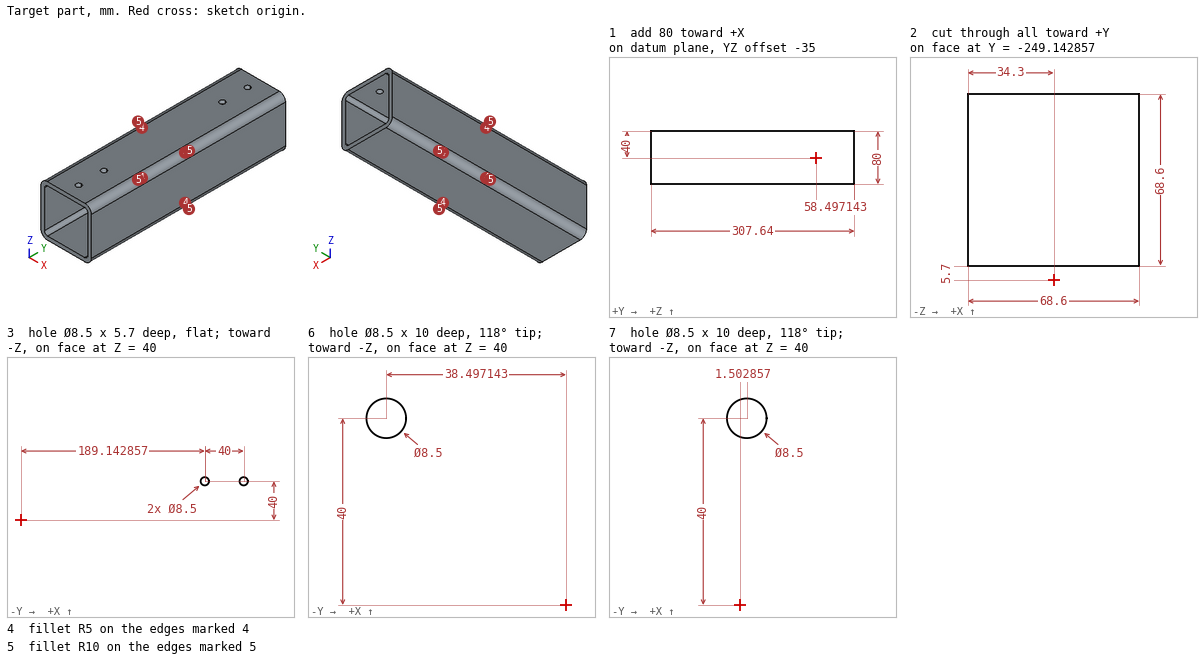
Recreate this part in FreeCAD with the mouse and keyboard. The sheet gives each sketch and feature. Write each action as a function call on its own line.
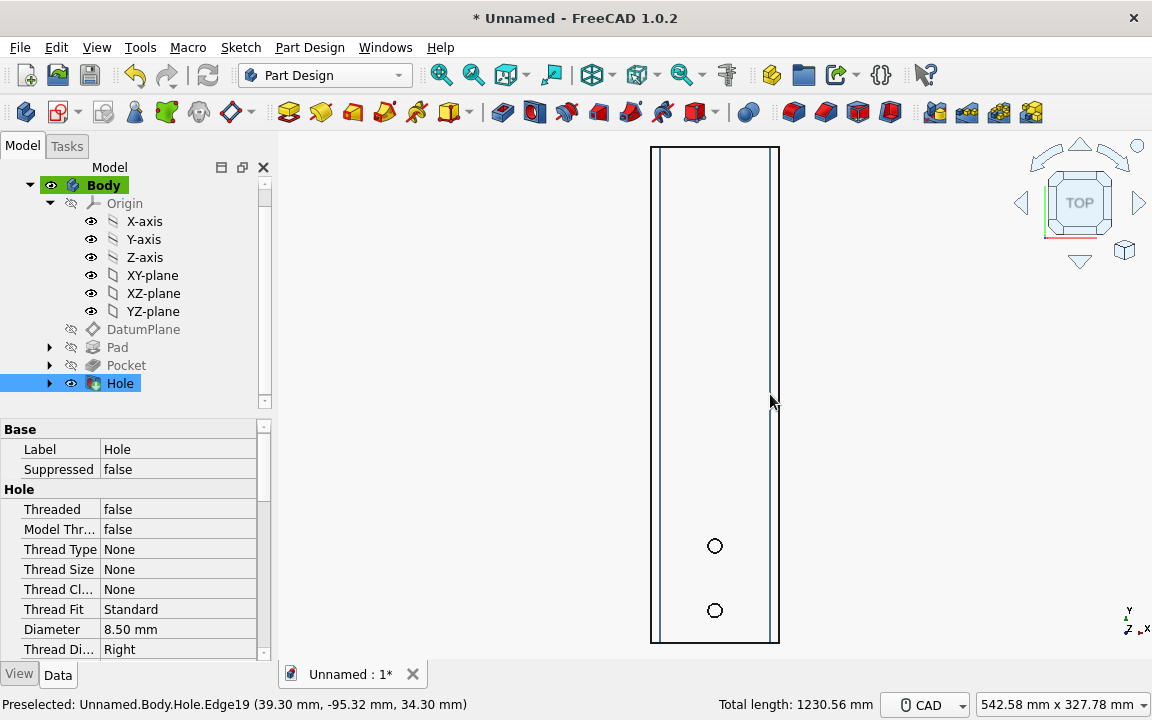
key(v)
key(1)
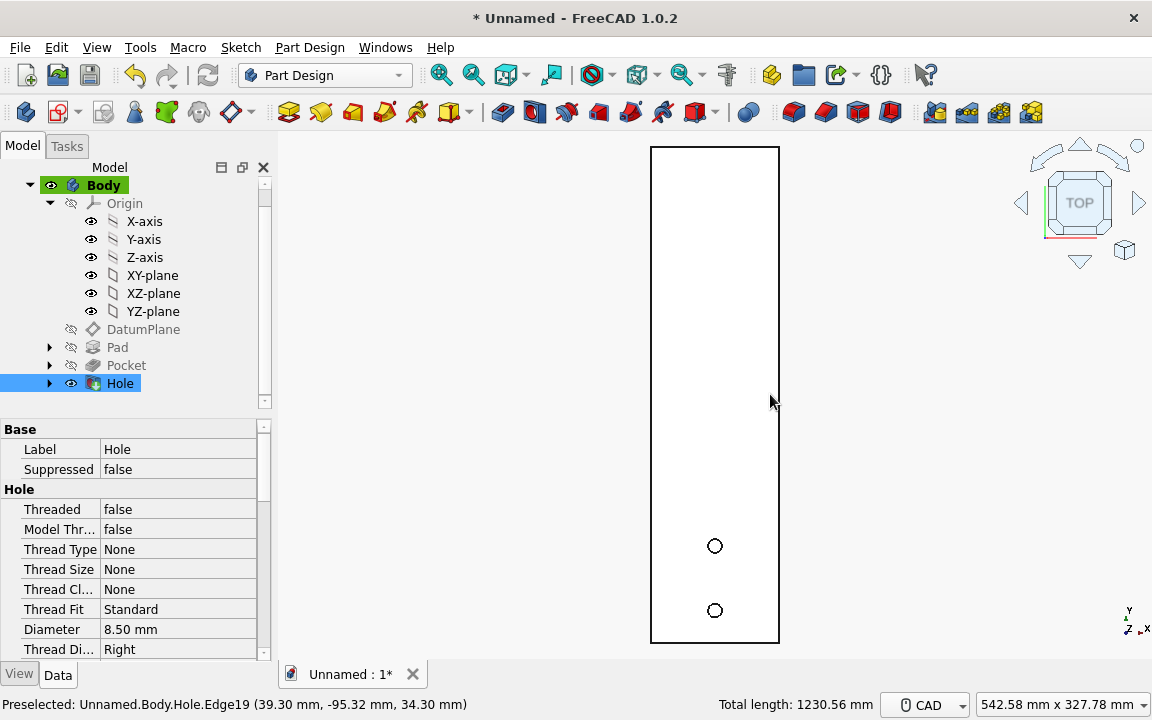
click(794, 112)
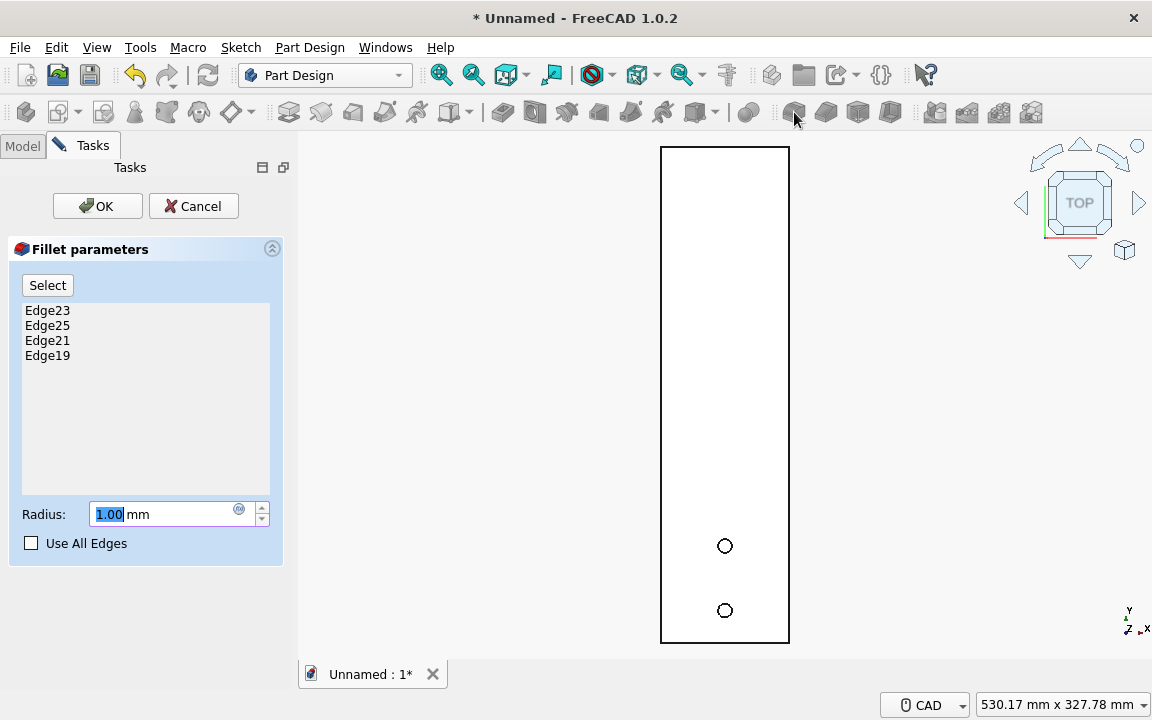
text(5)
key(Tab)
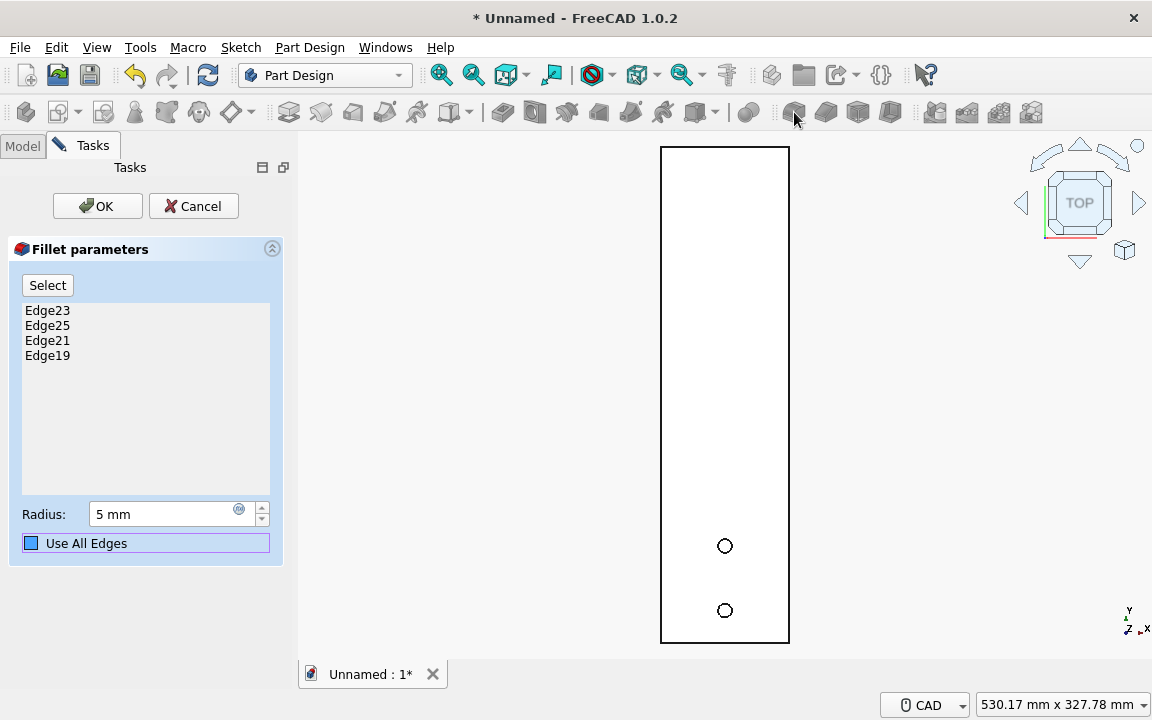
click(98, 206)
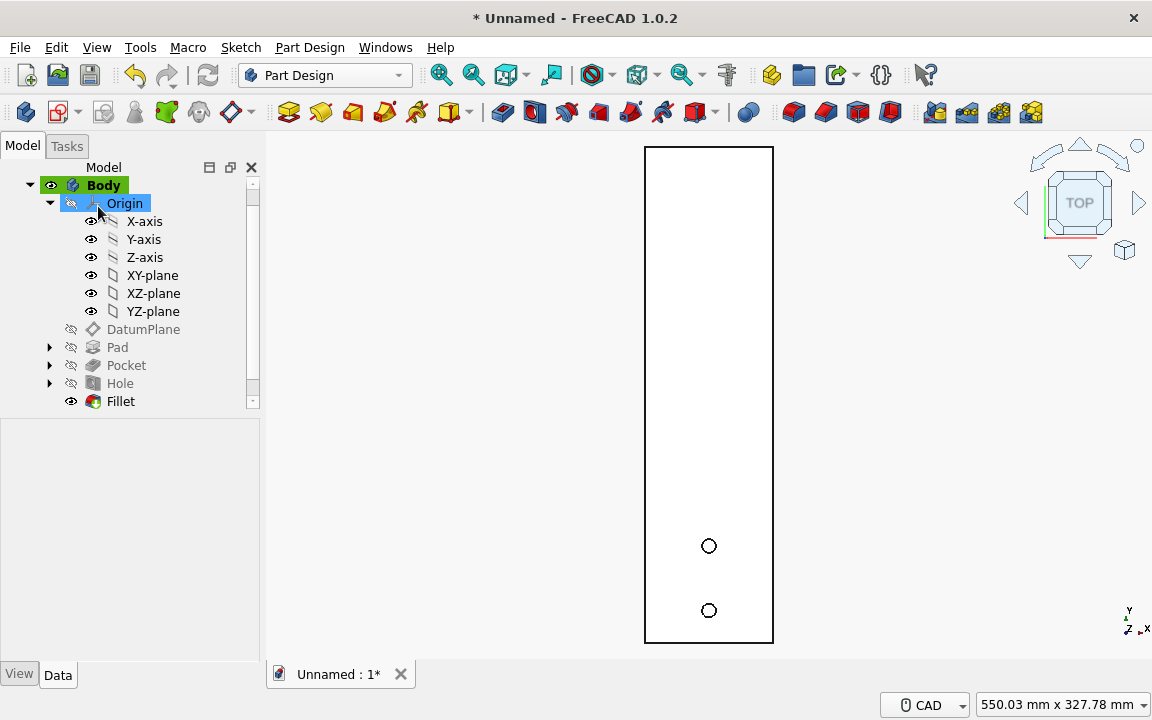
click(773, 394)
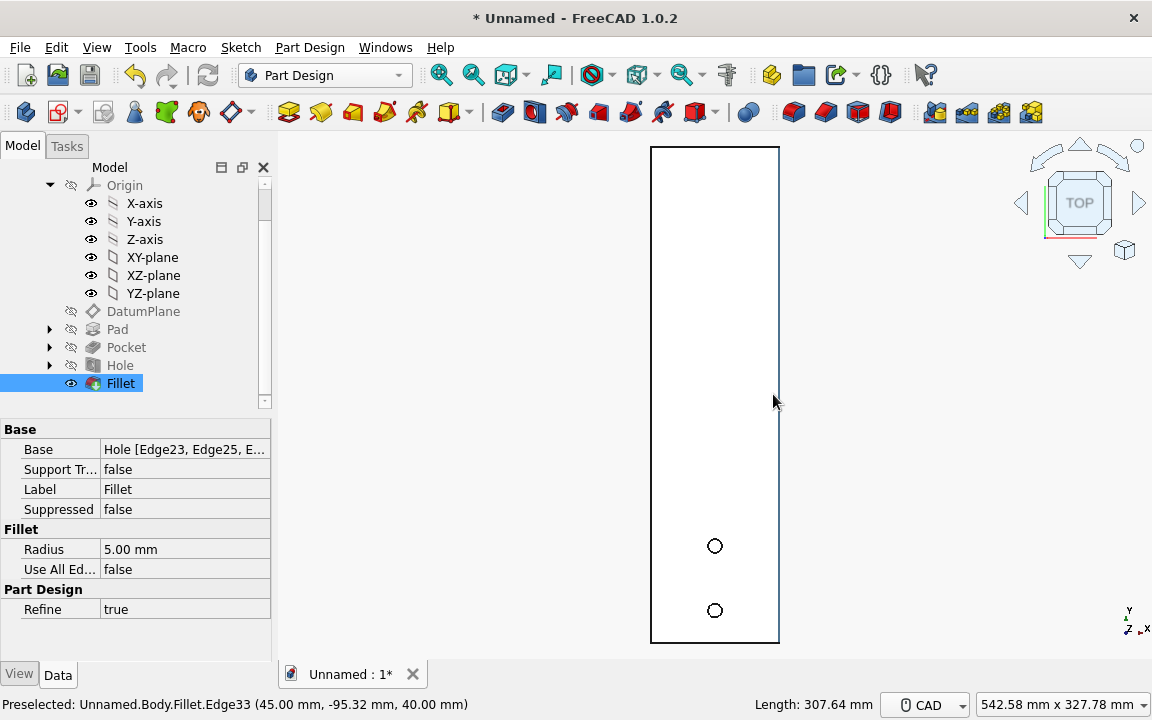
click(651, 394, ctrl)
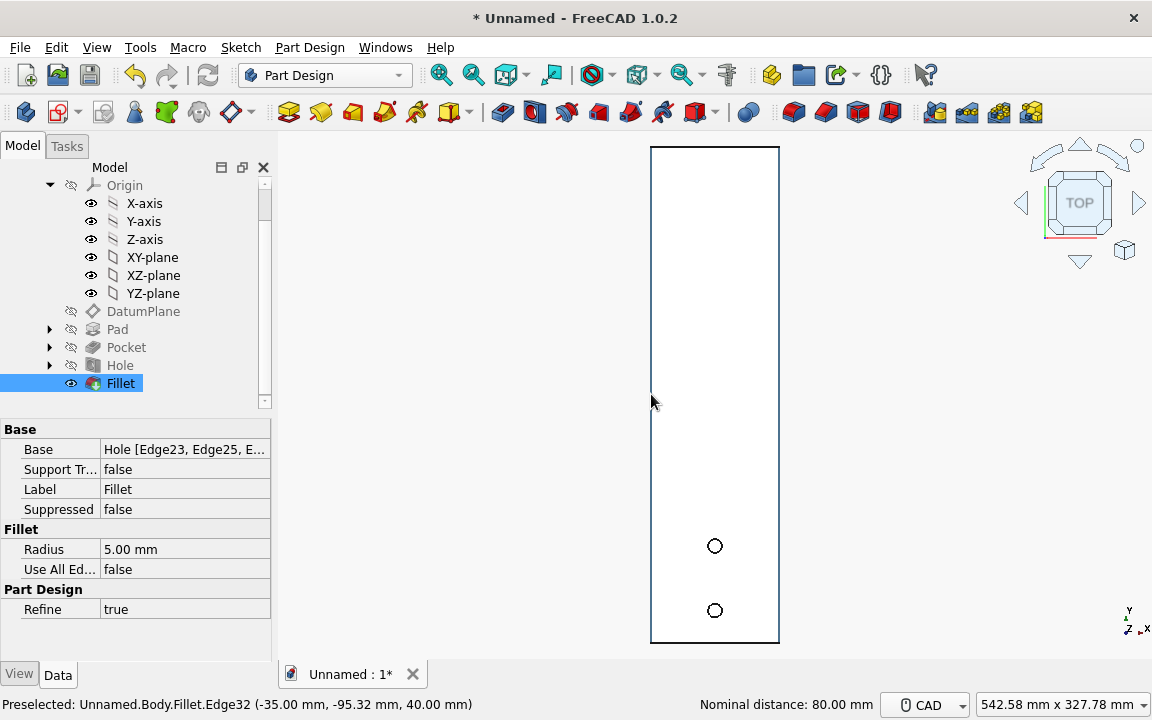
key(0)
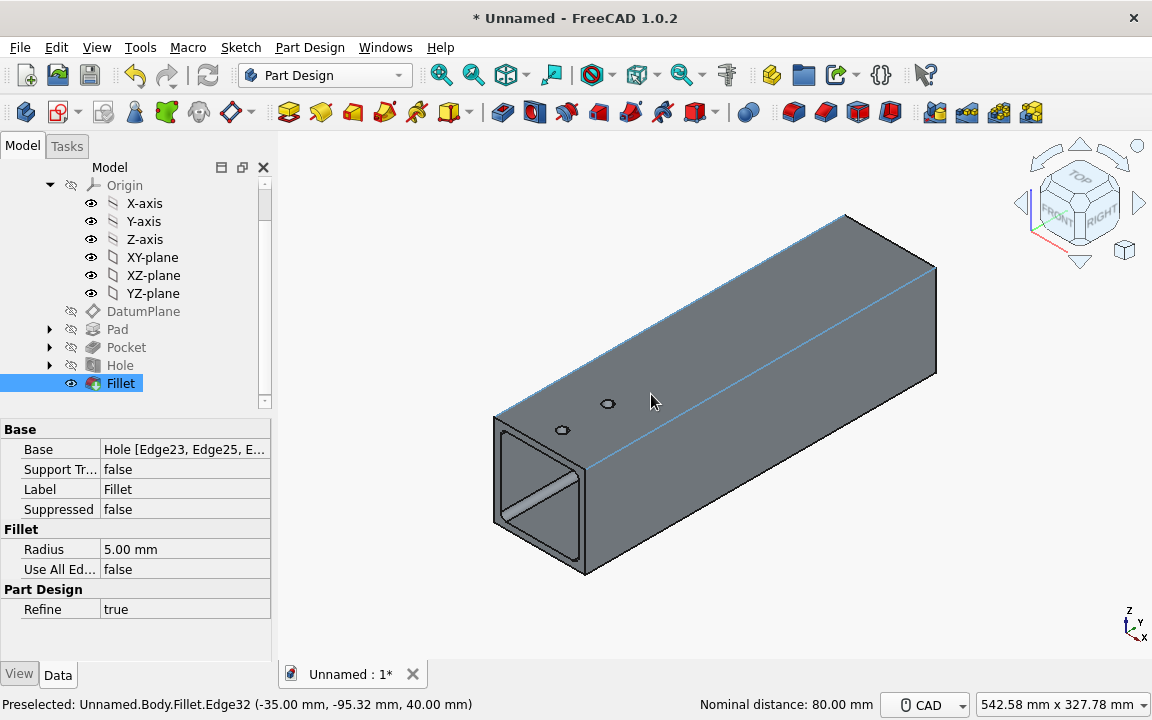
key(2)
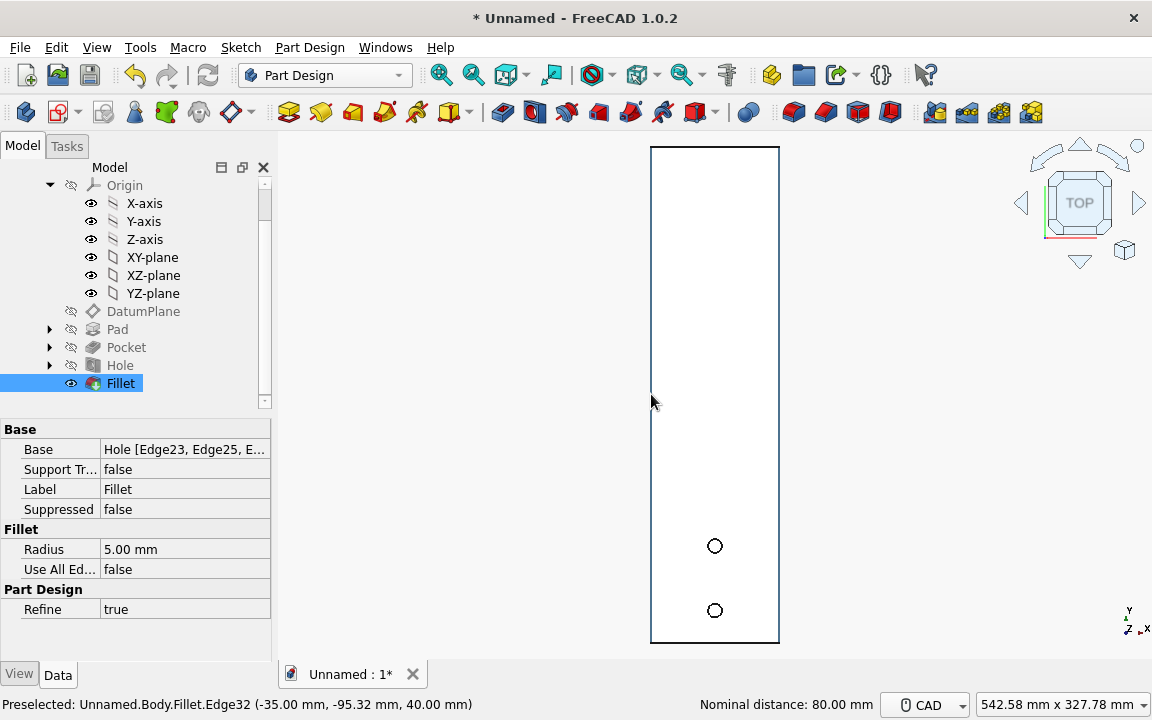
key(1)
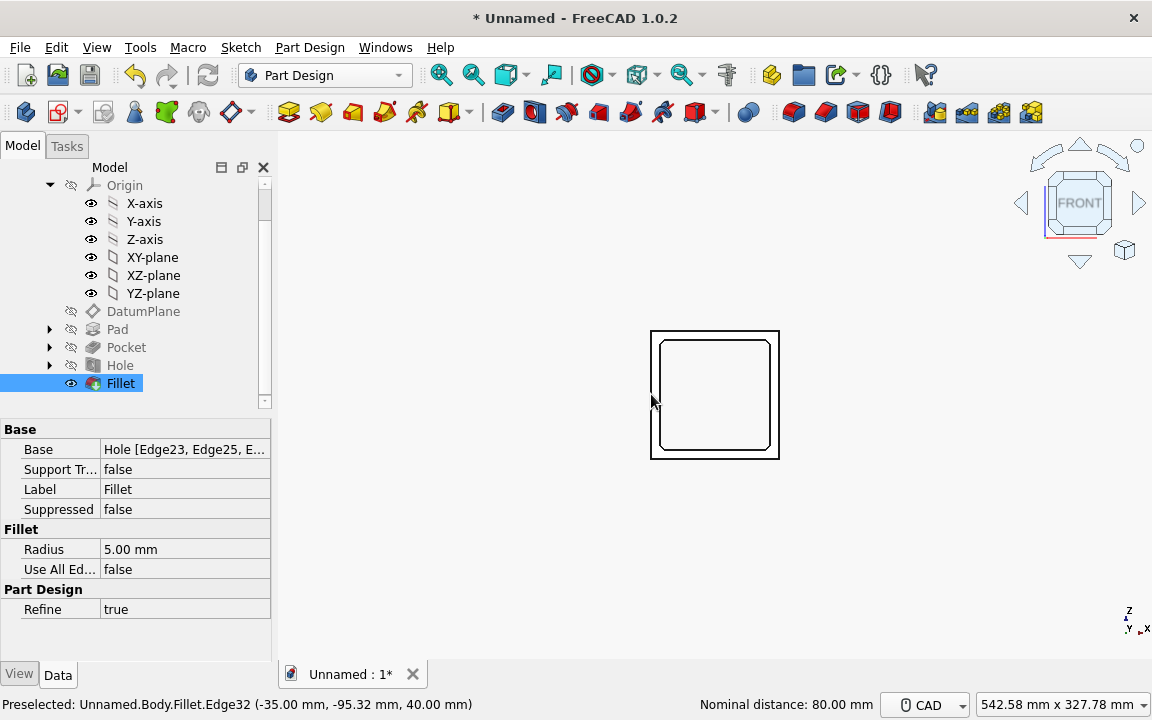
key(v)
key(f)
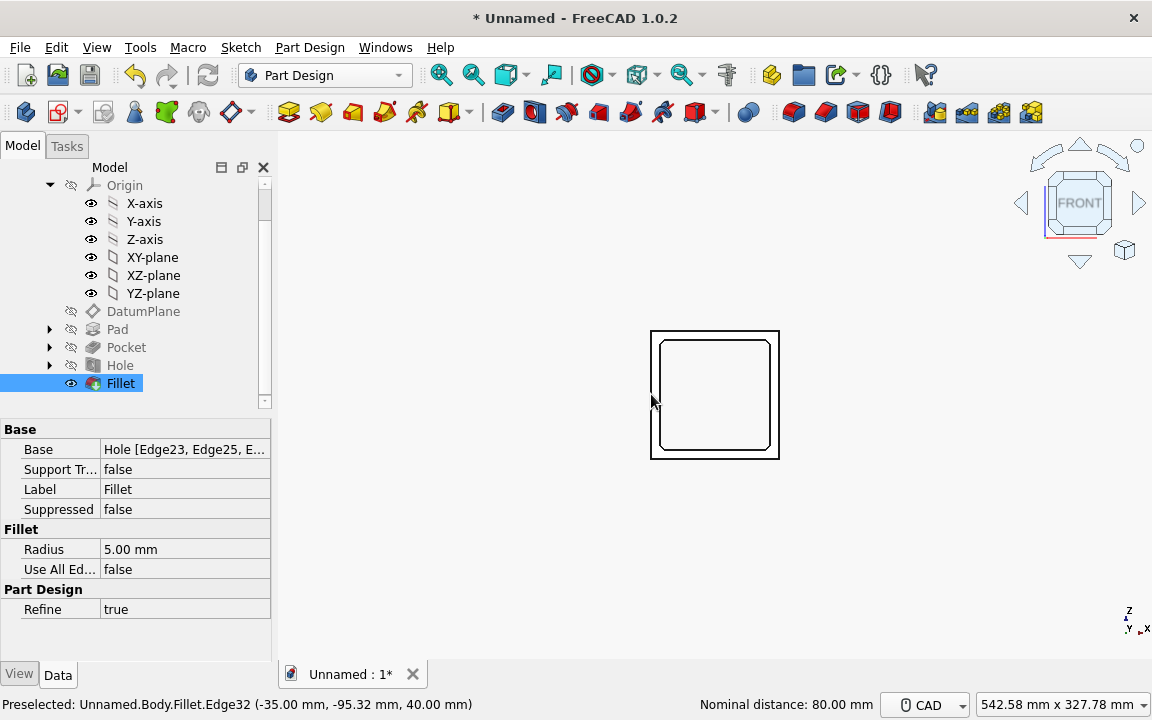
key(3)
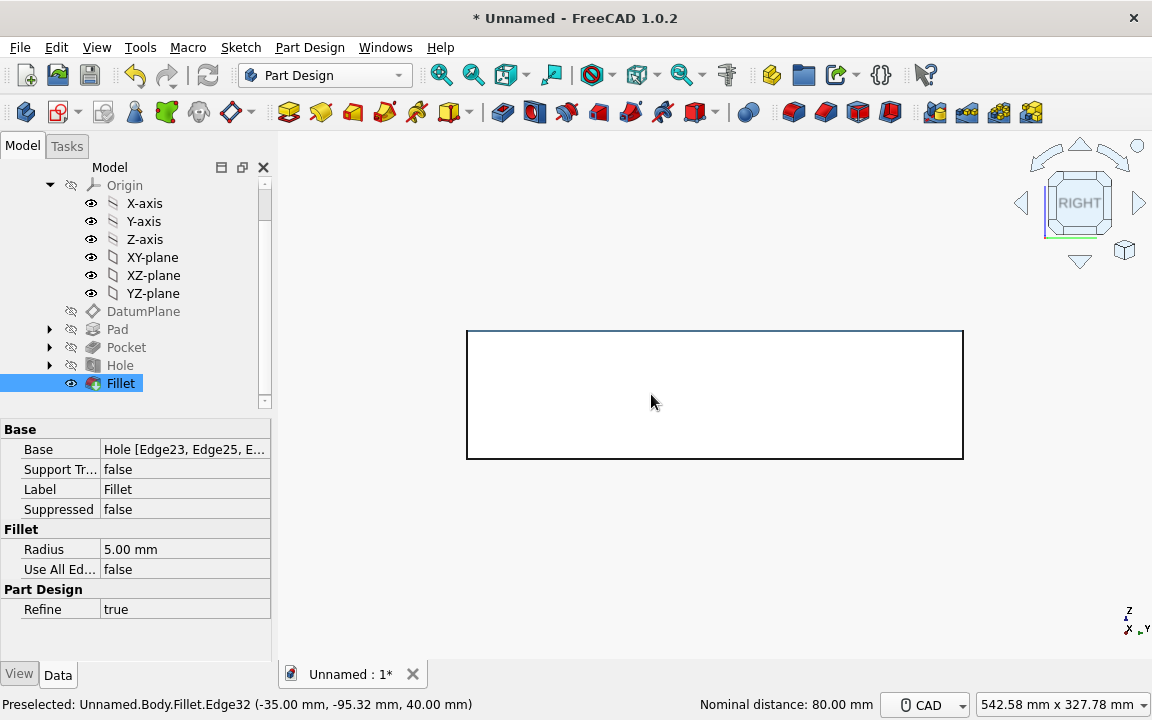
click(715, 458, ctrl)